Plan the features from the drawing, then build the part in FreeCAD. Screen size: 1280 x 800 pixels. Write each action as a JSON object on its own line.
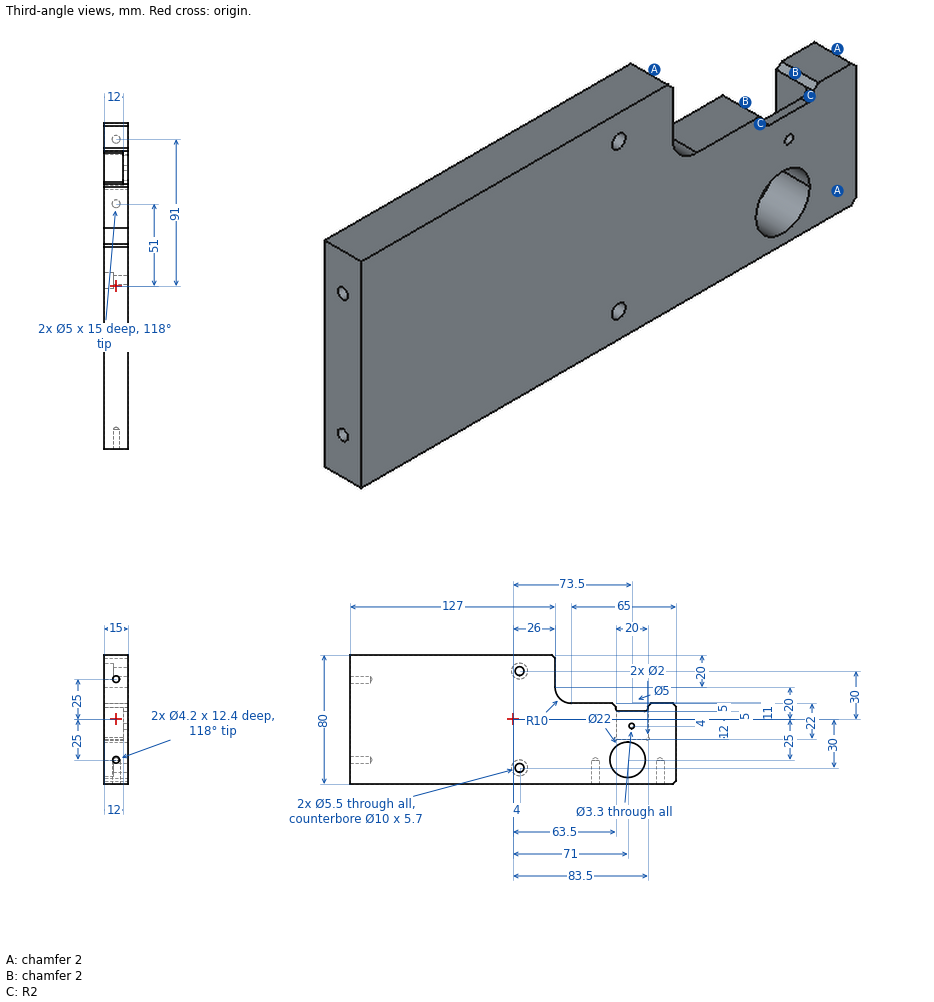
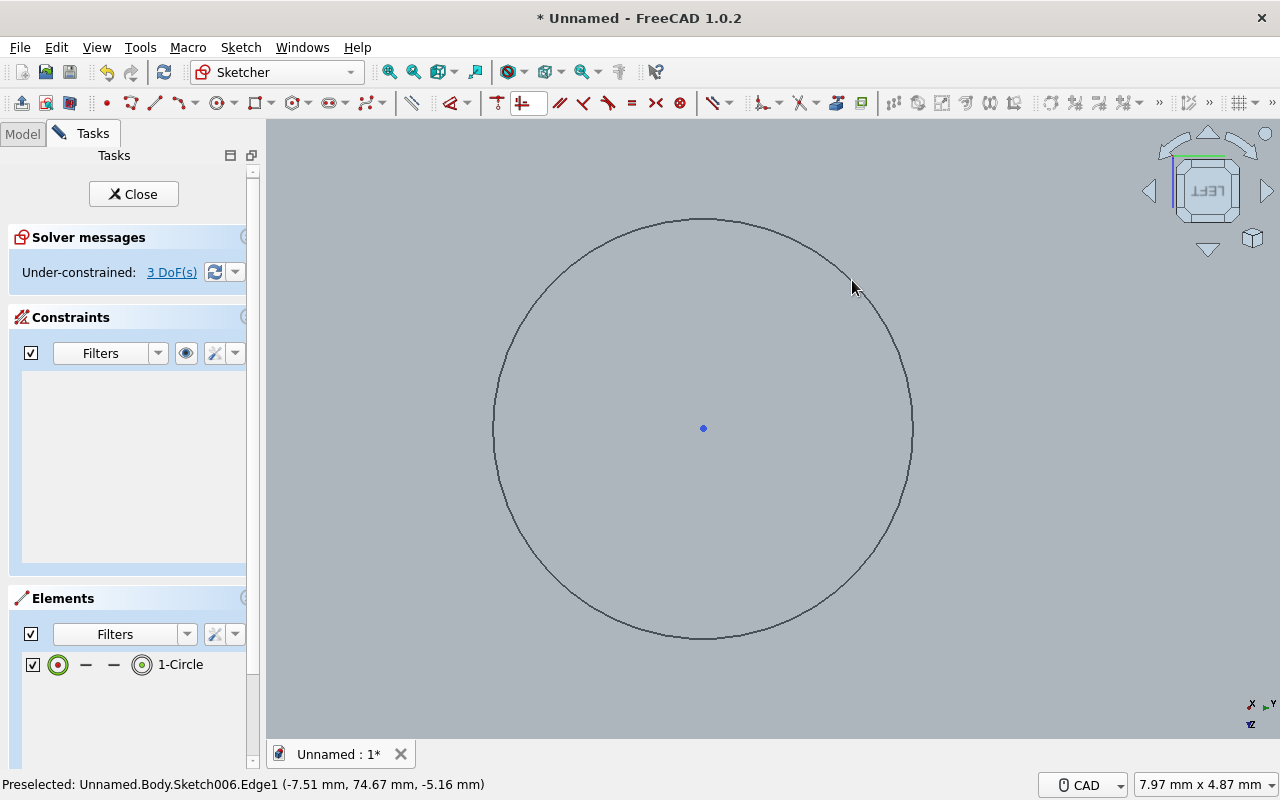
{"action": "left_click", "coordinate": [450, 104]}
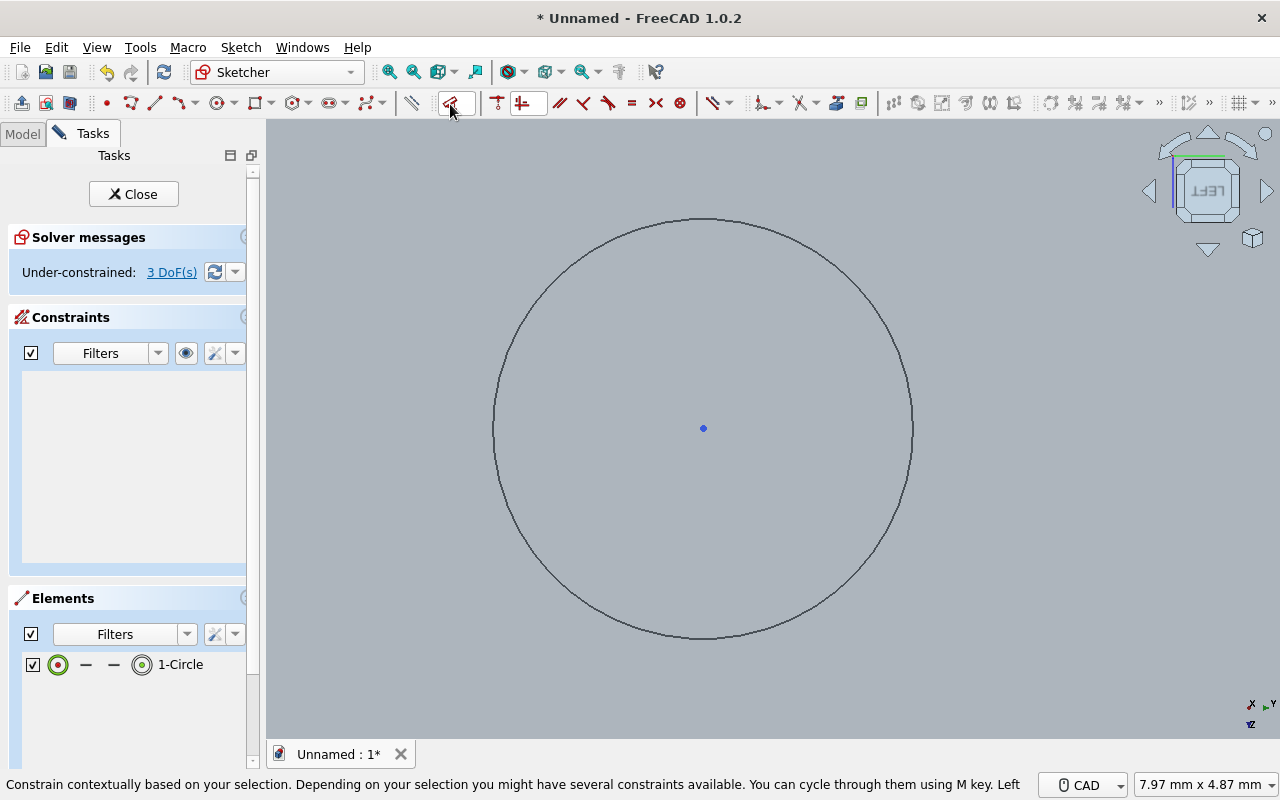
{"action": "left_click", "coordinate": [851, 280]}
{"action": "left_click", "coordinate": [874, 257]}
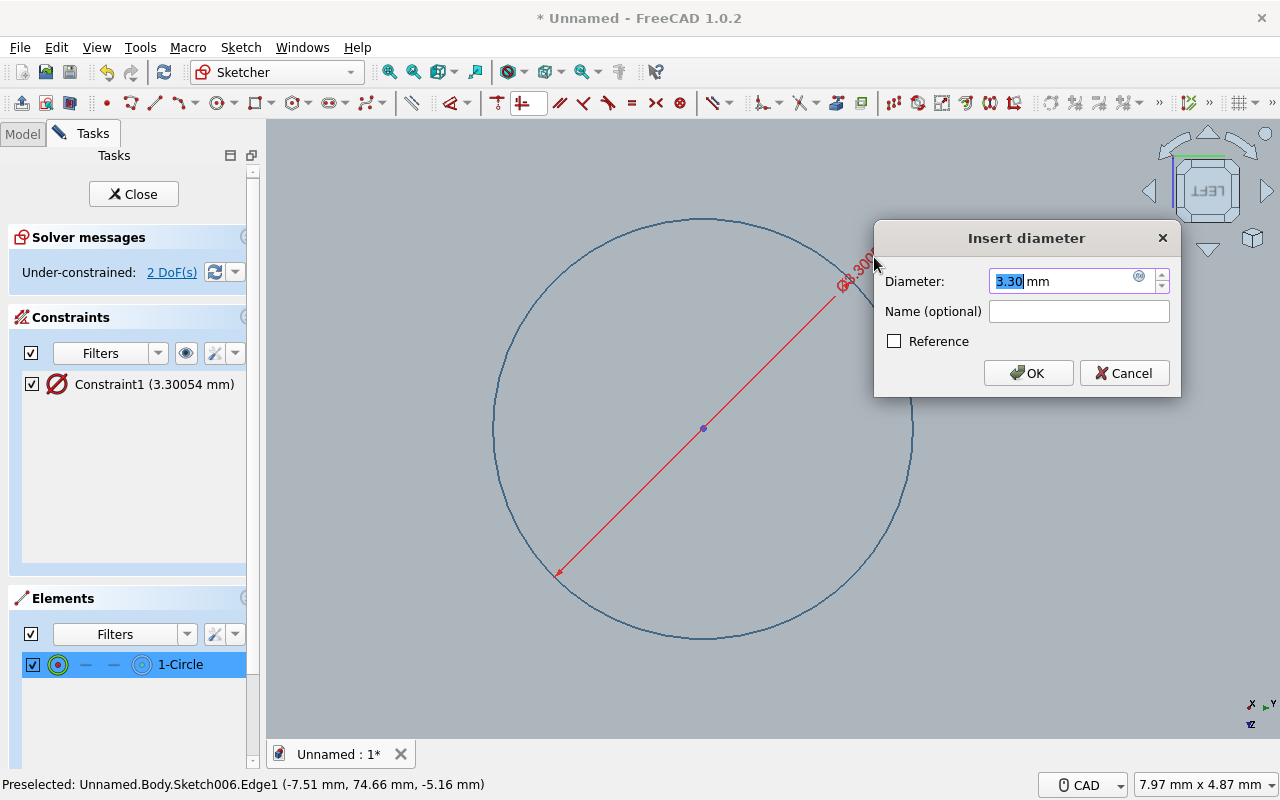
{"action": "type", "text": "3.3"}
{"action": "key", "text": "Return"}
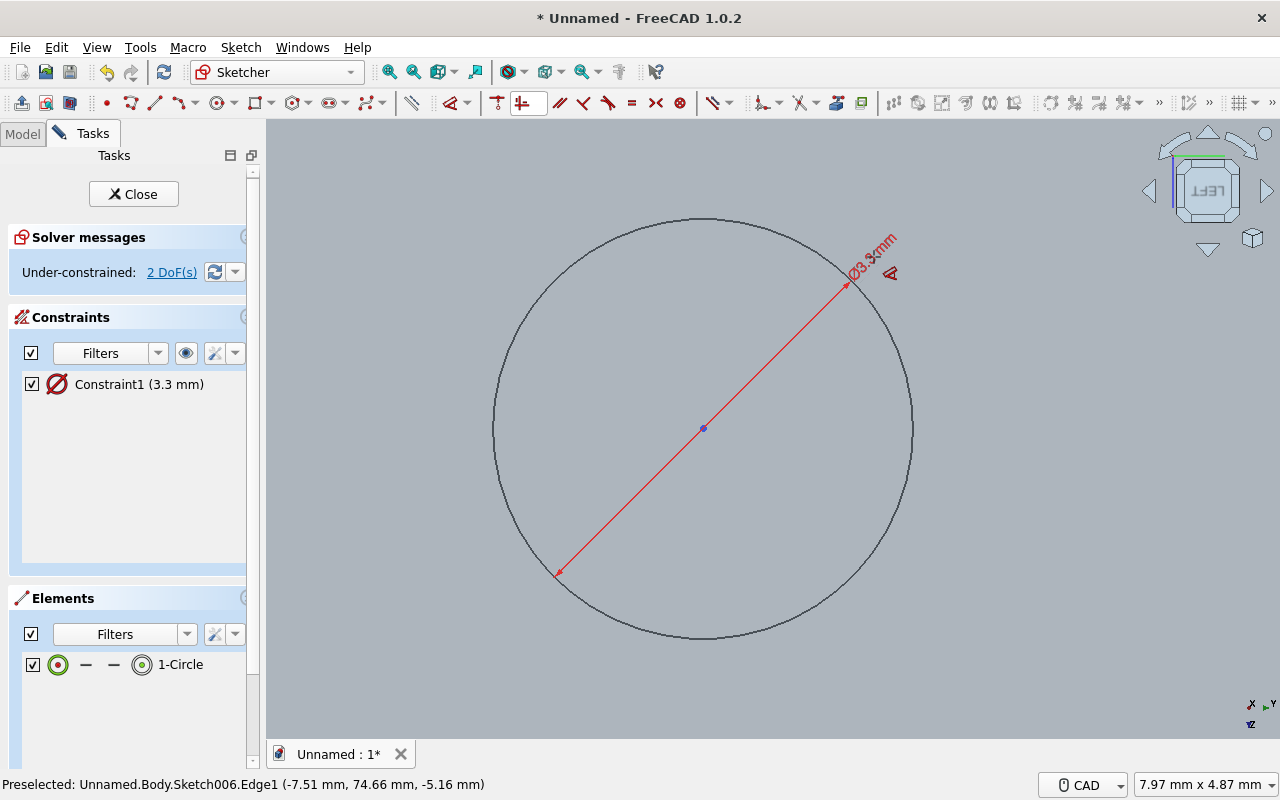
{"action": "left_click", "coordinate": [703, 429]}
{"action": "left_click", "coordinate": [737, 570]}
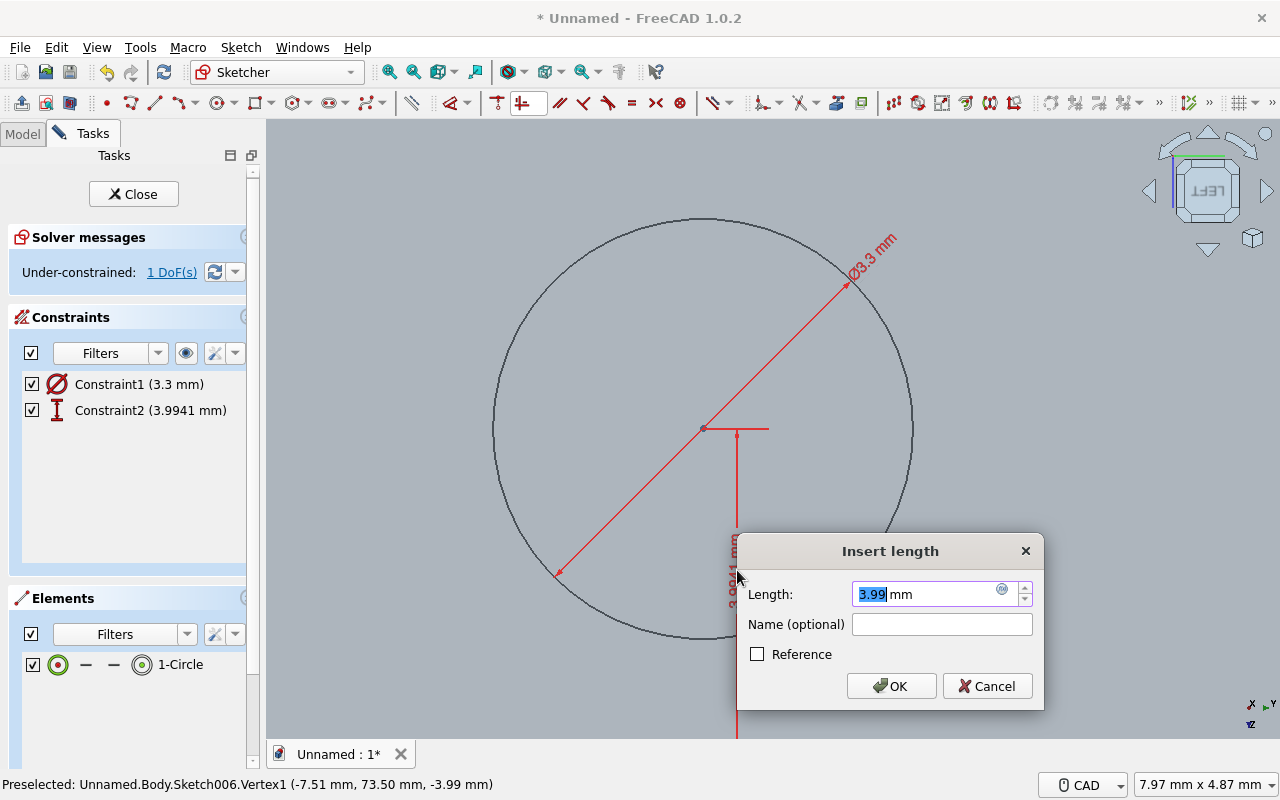
{"action": "type", "text": "4"}
{"action": "key", "text": "Return"}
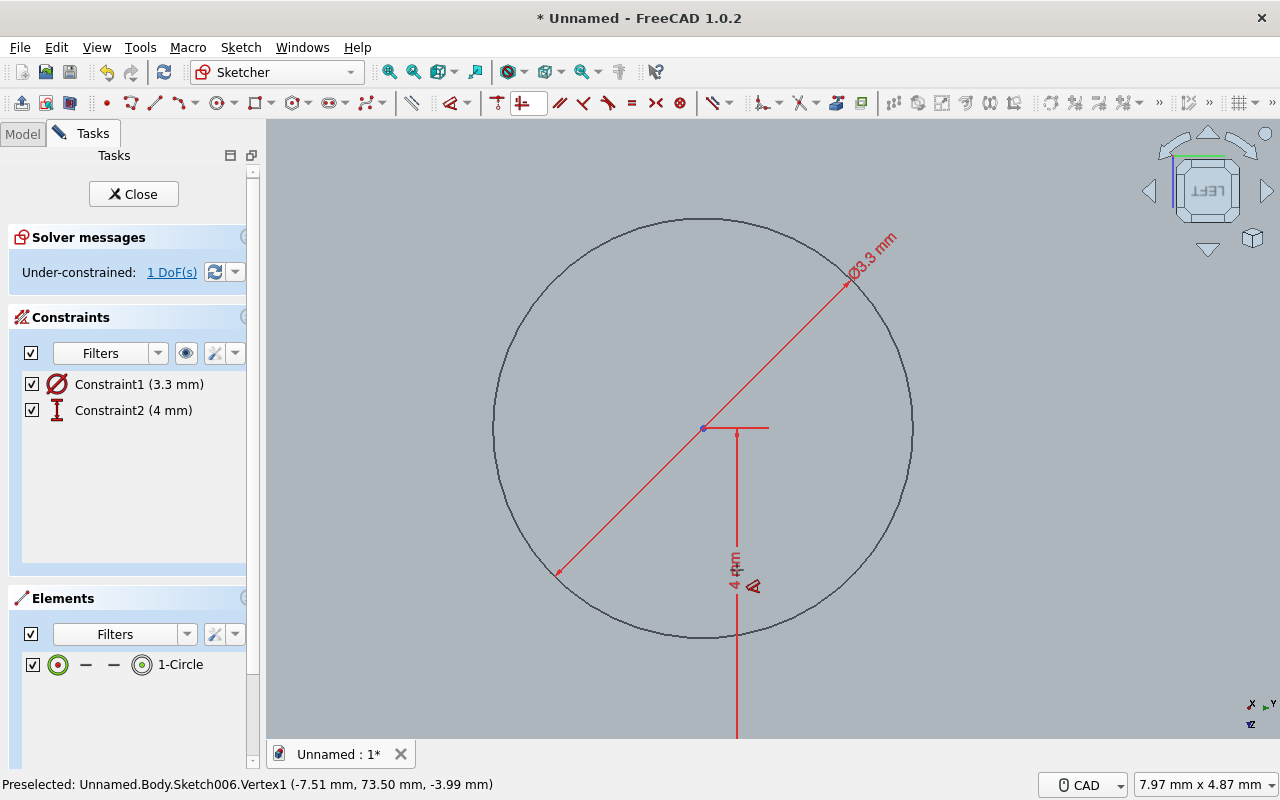
{"action": "left_click", "coordinate": [703, 428]}
{"action": "left_click", "coordinate": [404, 394]}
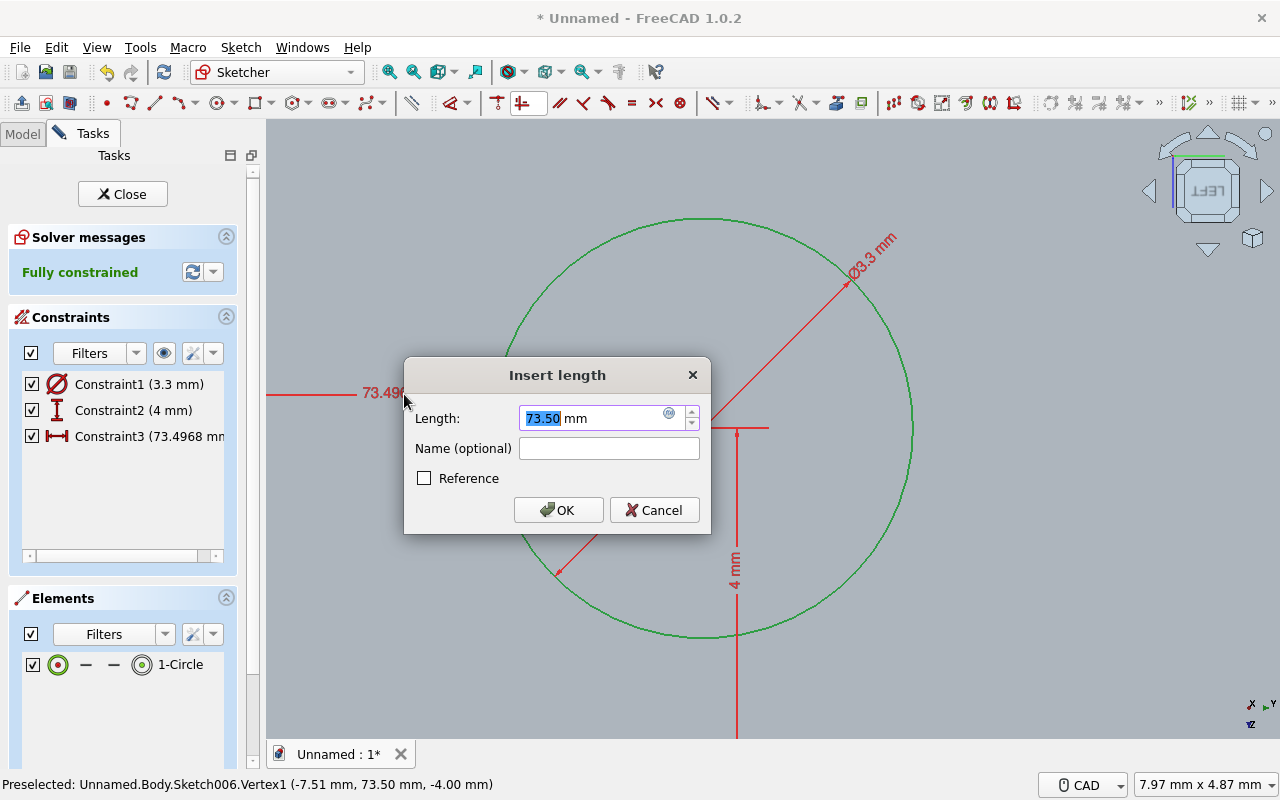
{"action": "type", "text": "73.5"}
{"action": "key", "text": "Return"}
{"action": "key", "text": "Escape"}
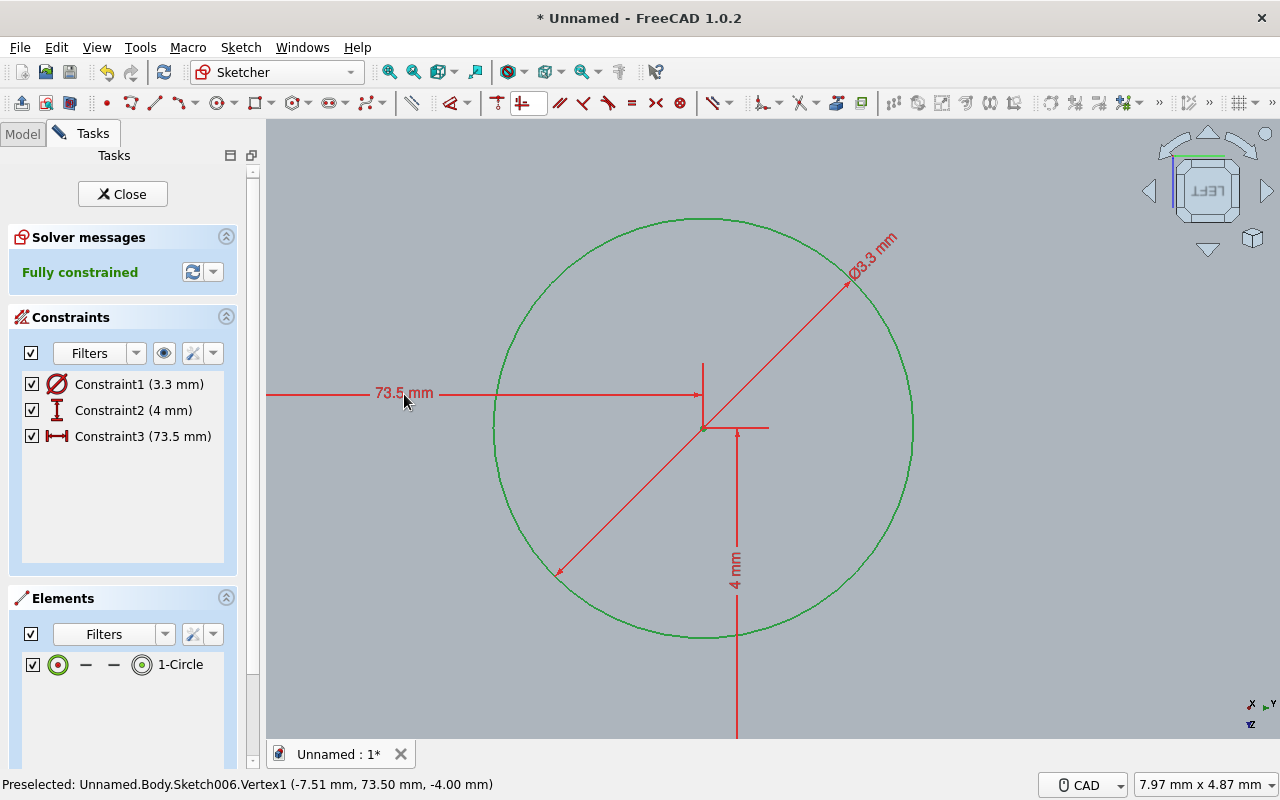
{"action": "left_click", "coordinate": [123, 194]}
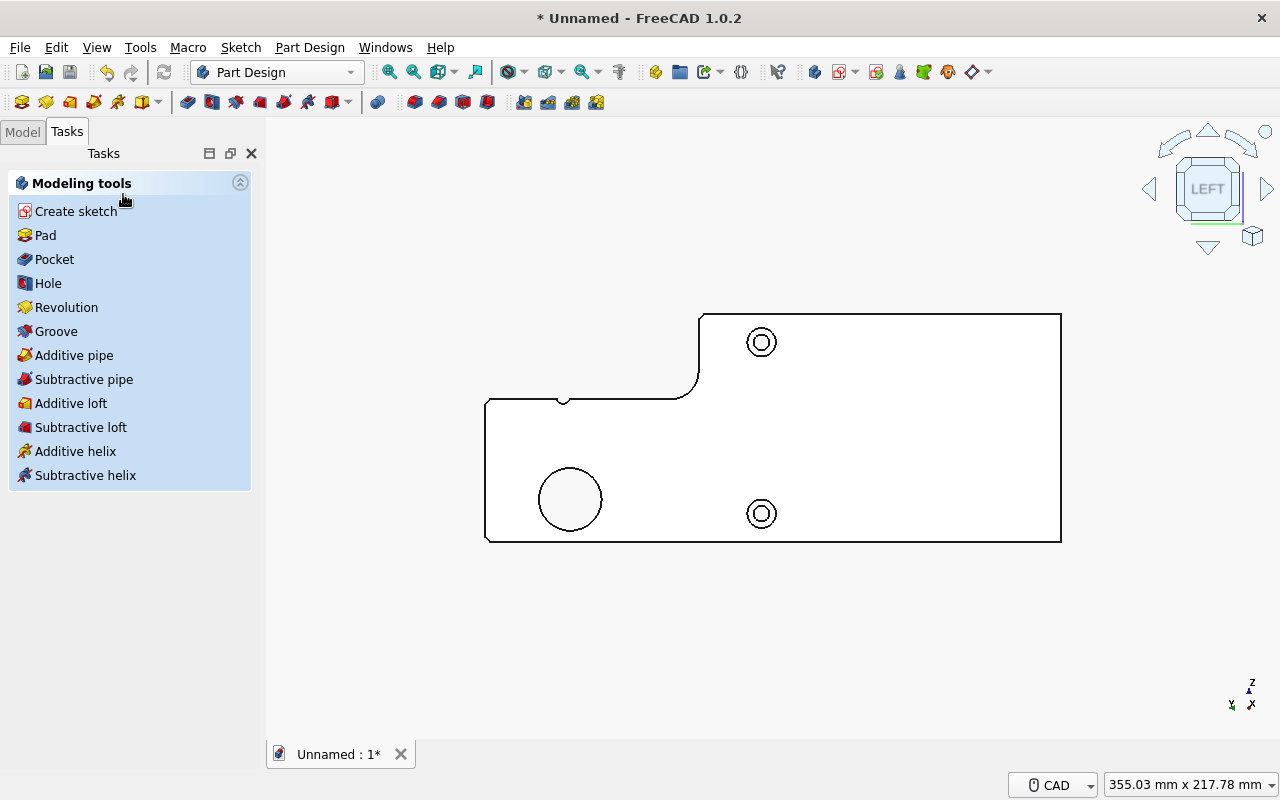
{"action": "left_click", "coordinate": [212, 102]}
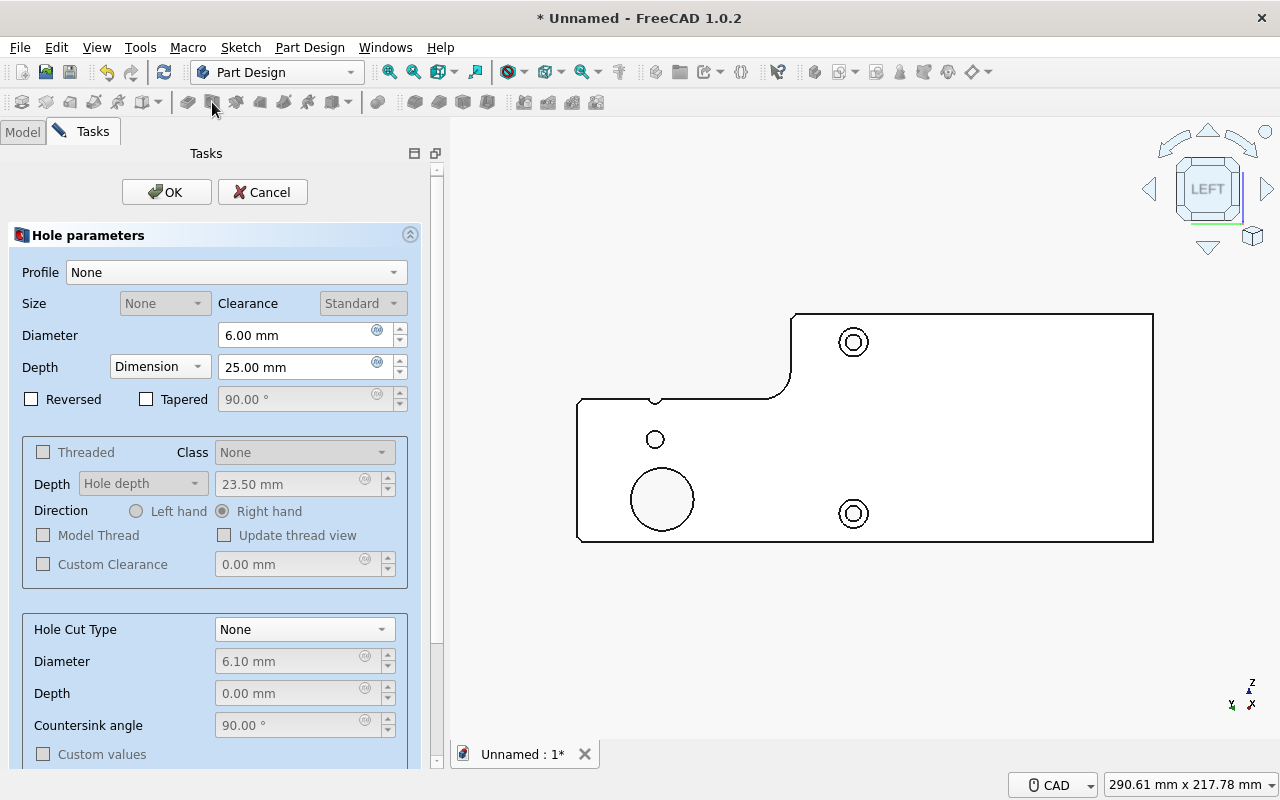
{"action": "triple_click", "coordinate": [305, 335]}